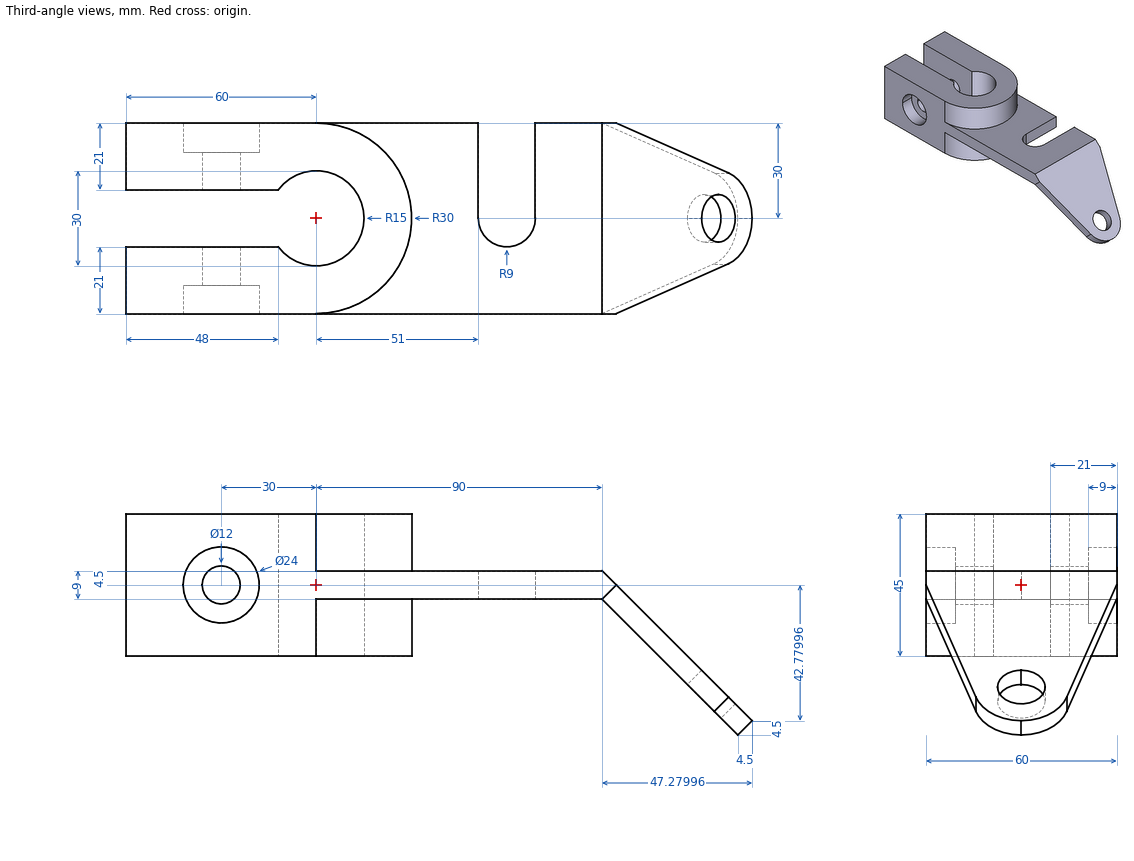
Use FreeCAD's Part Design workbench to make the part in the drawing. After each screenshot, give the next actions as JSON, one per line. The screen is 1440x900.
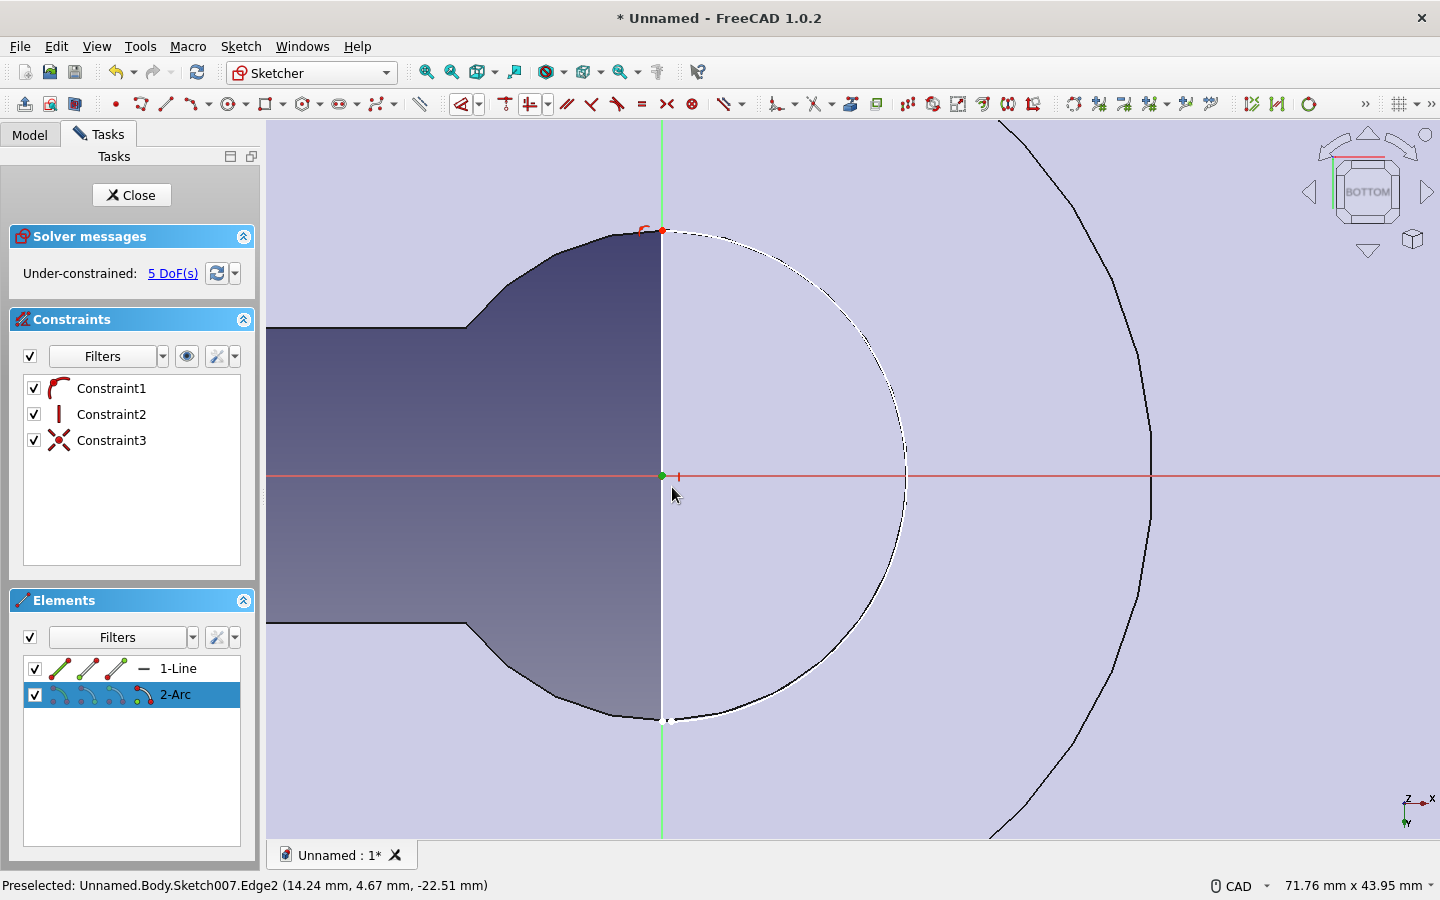
{"action": "left_click", "coordinate": [505, 104]}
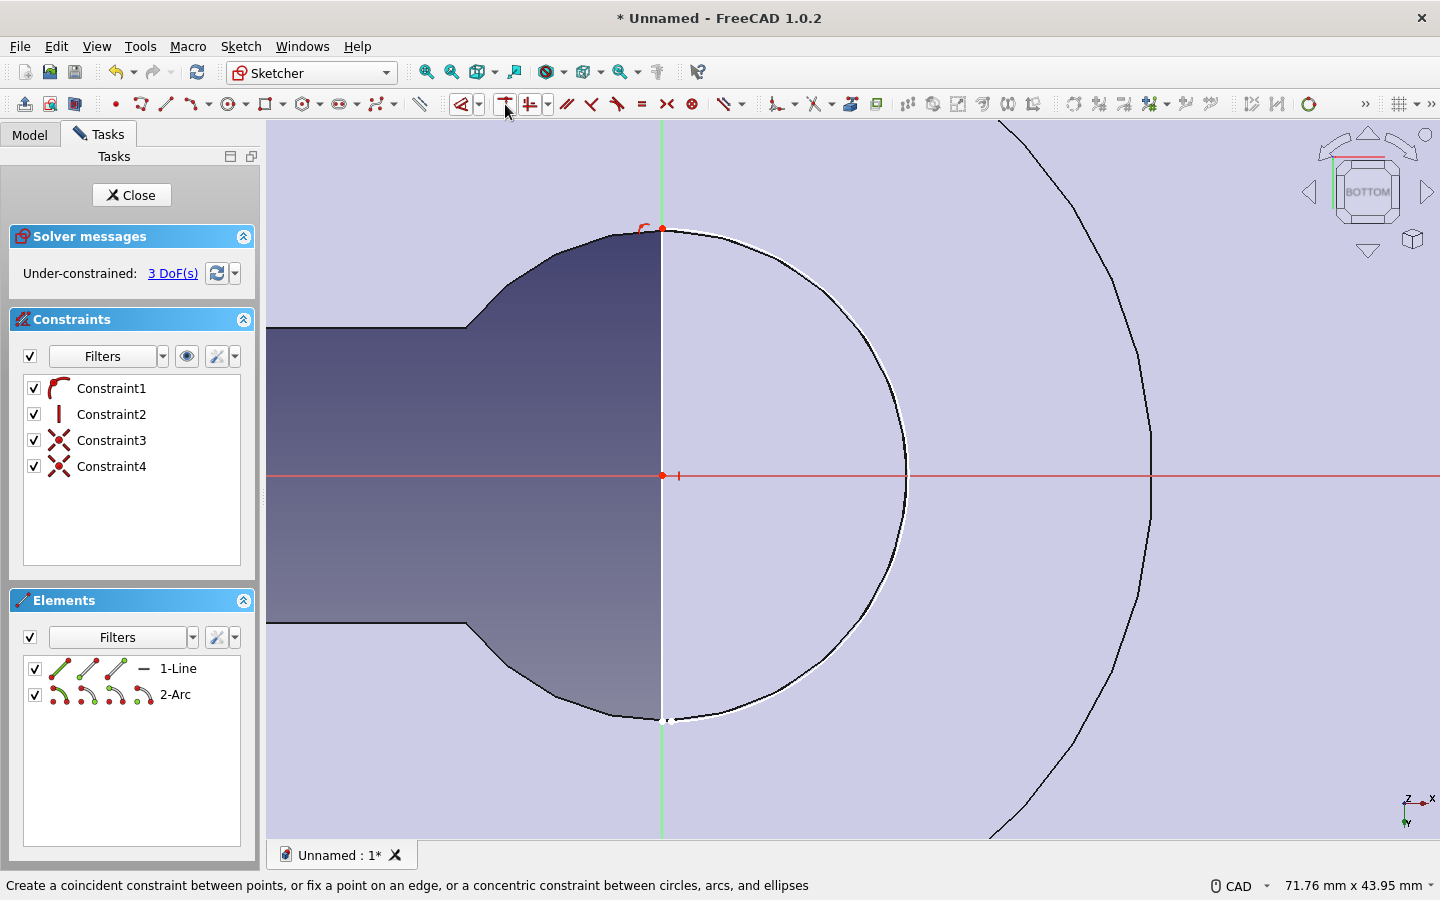
{"action": "left_click", "coordinate": [865, 615]}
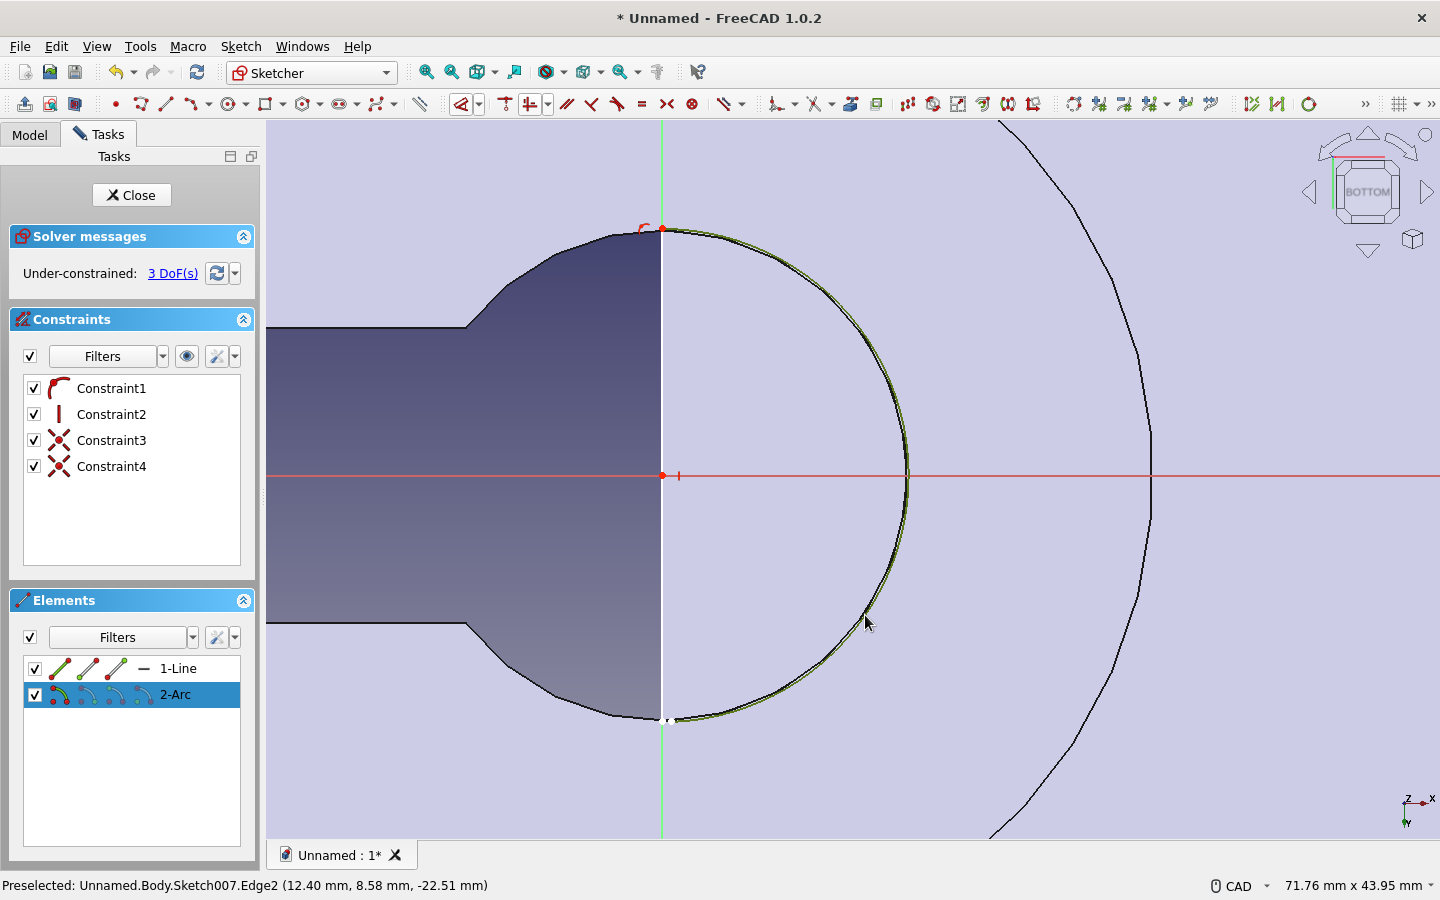
{"action": "left_click", "coordinate": [478, 104]}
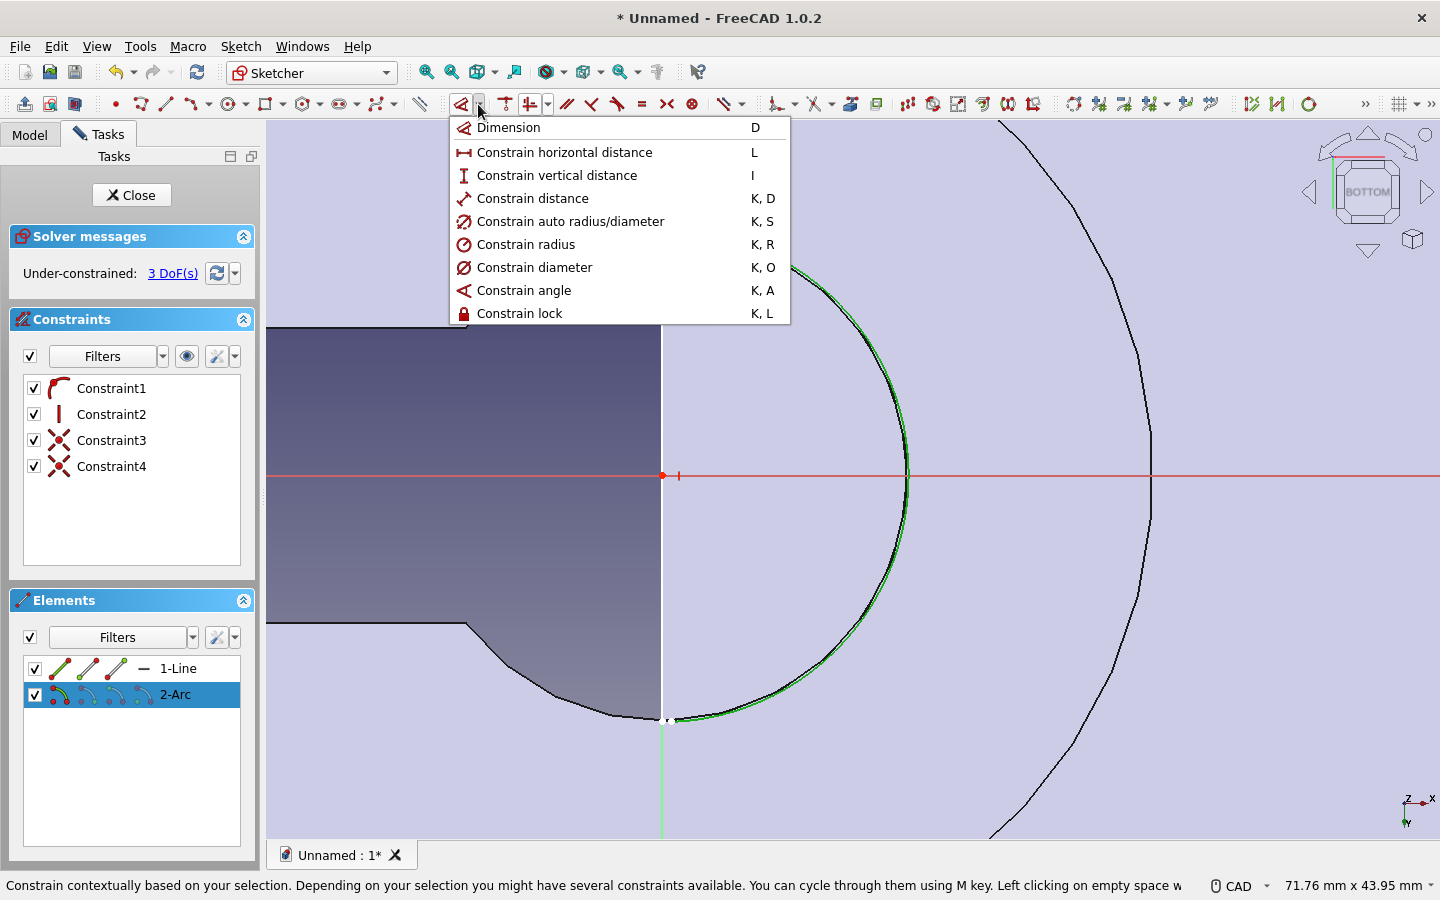
{"action": "left_click", "coordinate": [620, 244]}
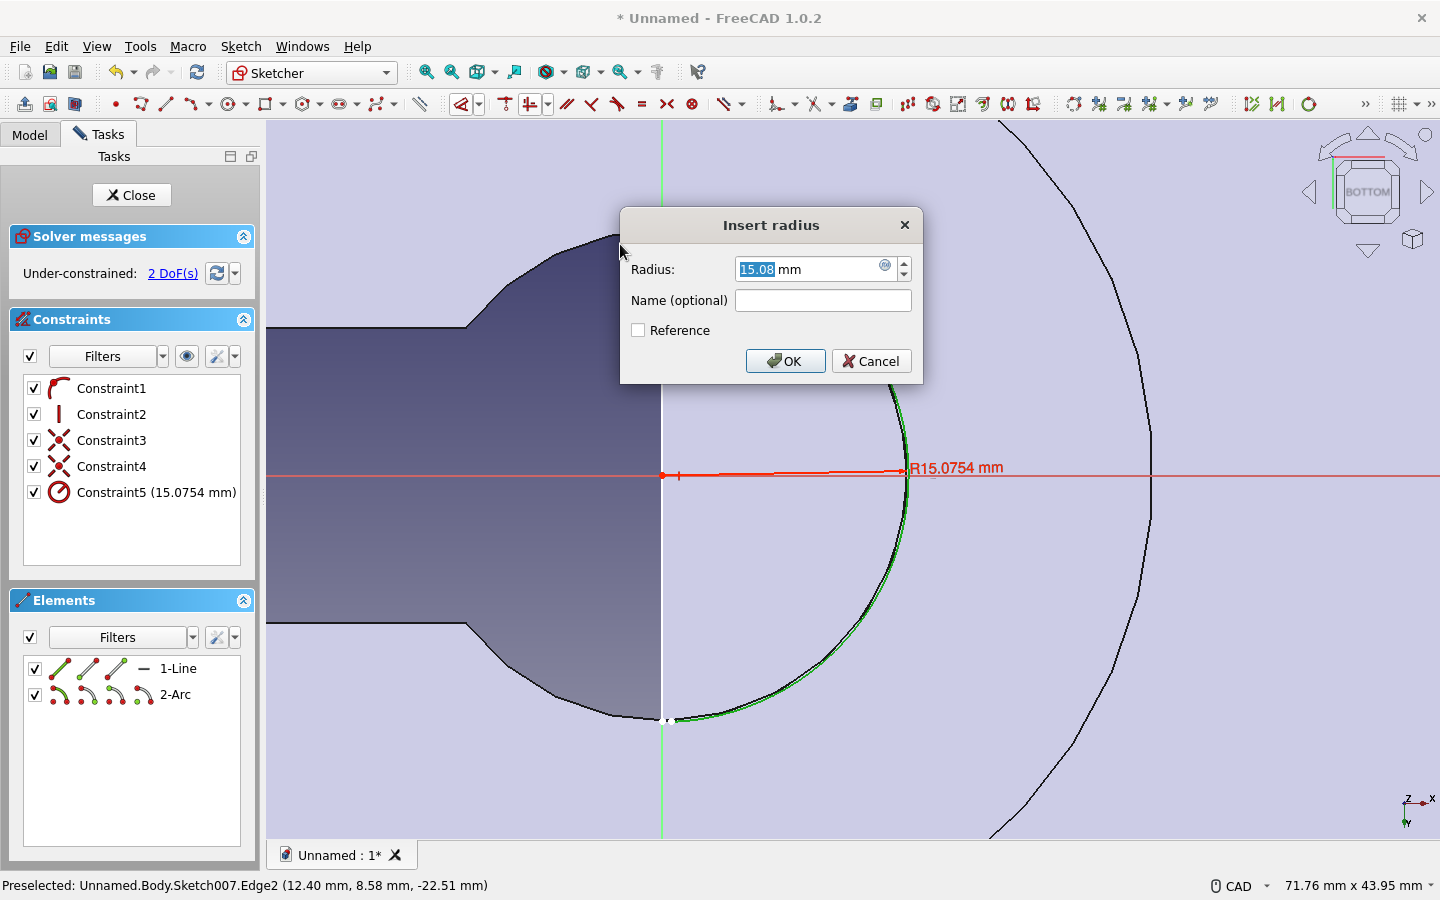
{"action": "type", "text": "15"}
{"action": "key", "text": "Return"}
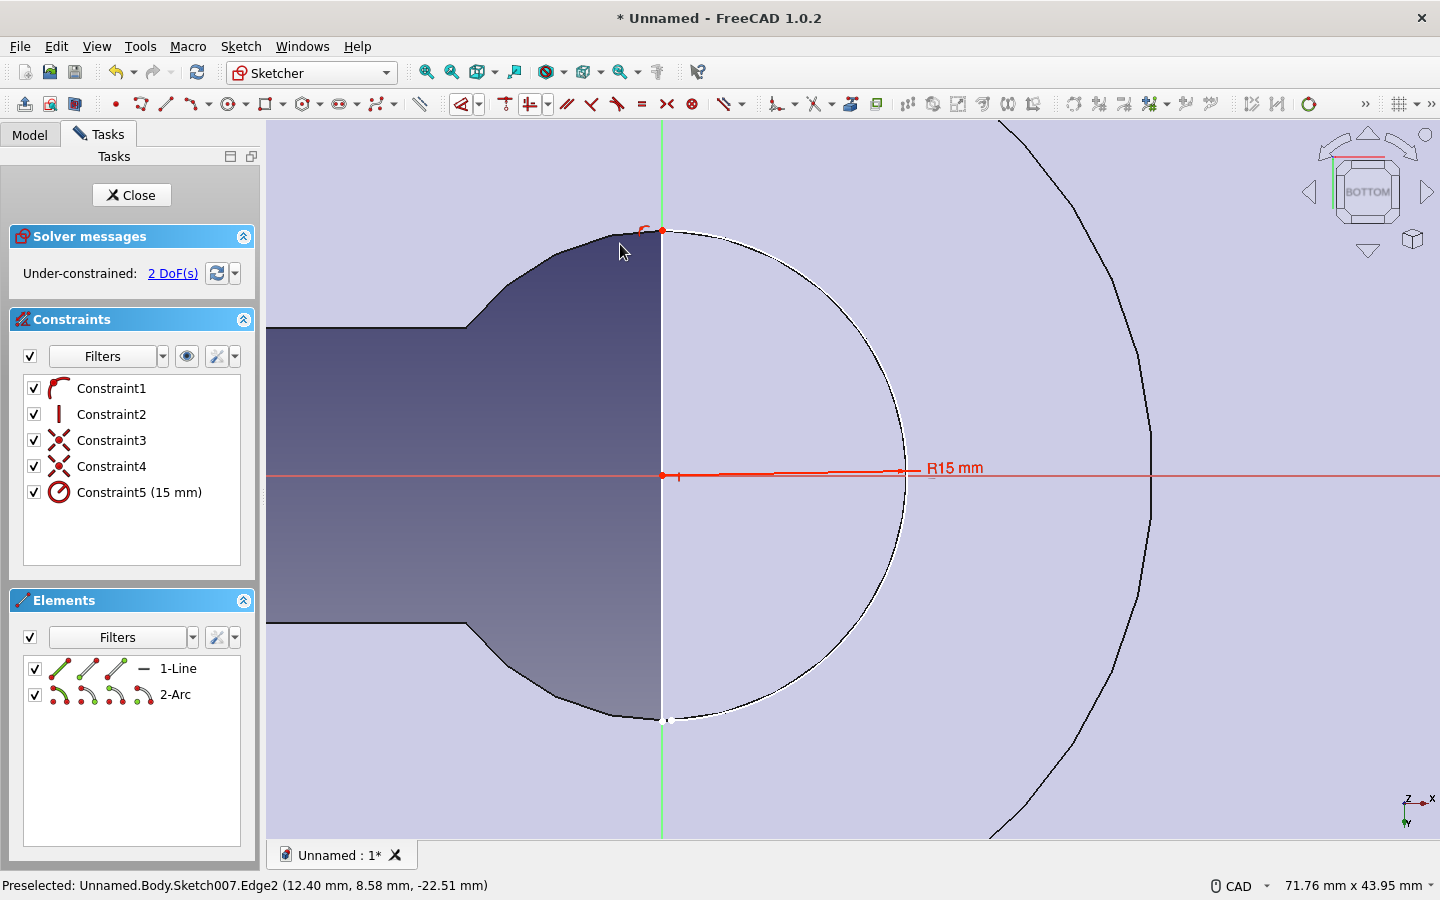
{"action": "left_click", "coordinate": [671, 721]}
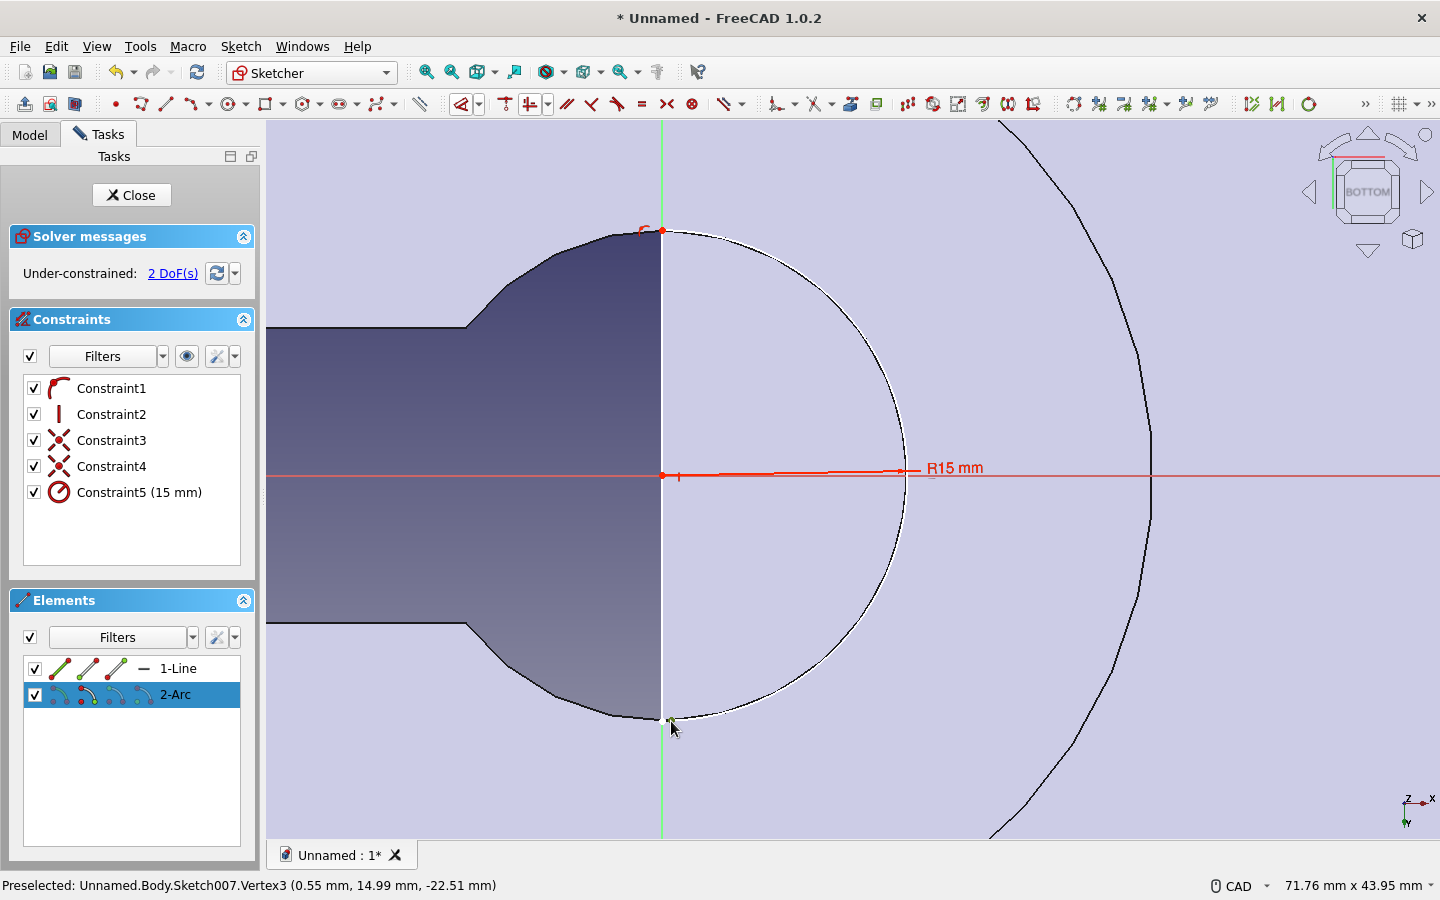
{"action": "left_click", "coordinate": [662, 764]}